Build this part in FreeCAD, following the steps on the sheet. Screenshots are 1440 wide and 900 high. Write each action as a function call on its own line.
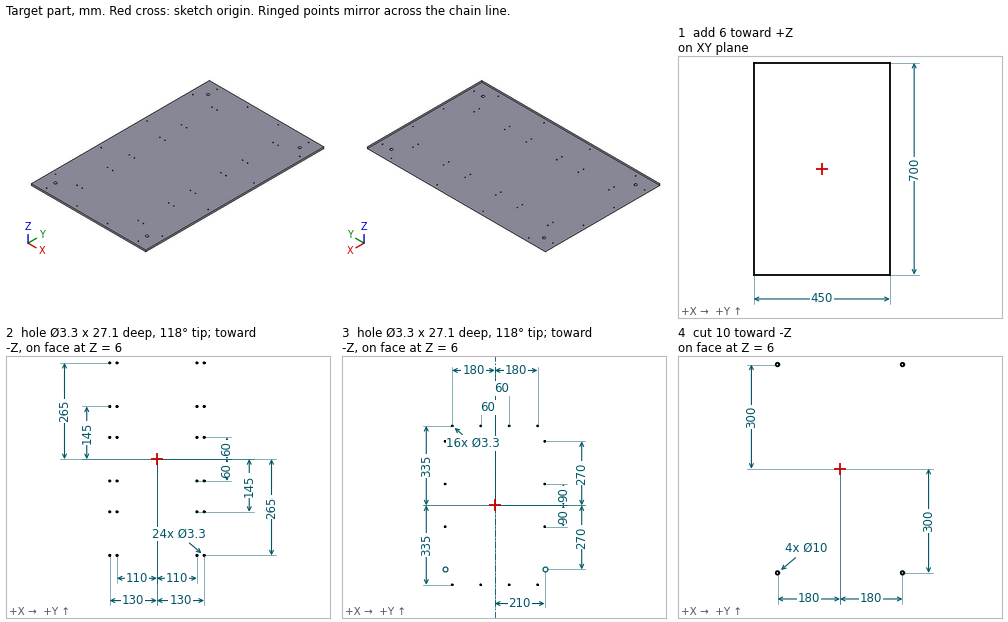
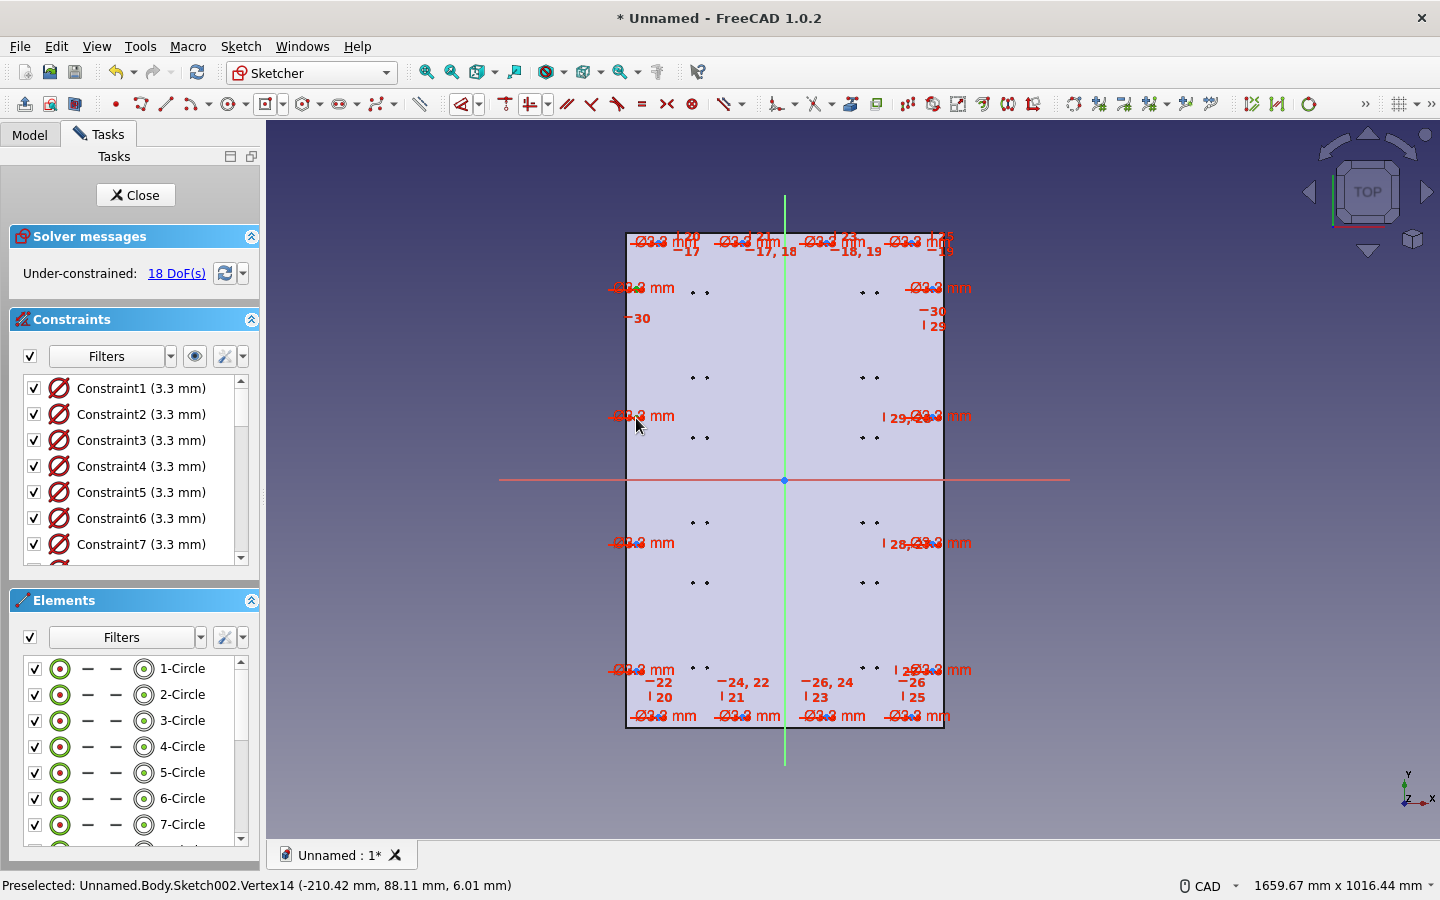
click(548, 104)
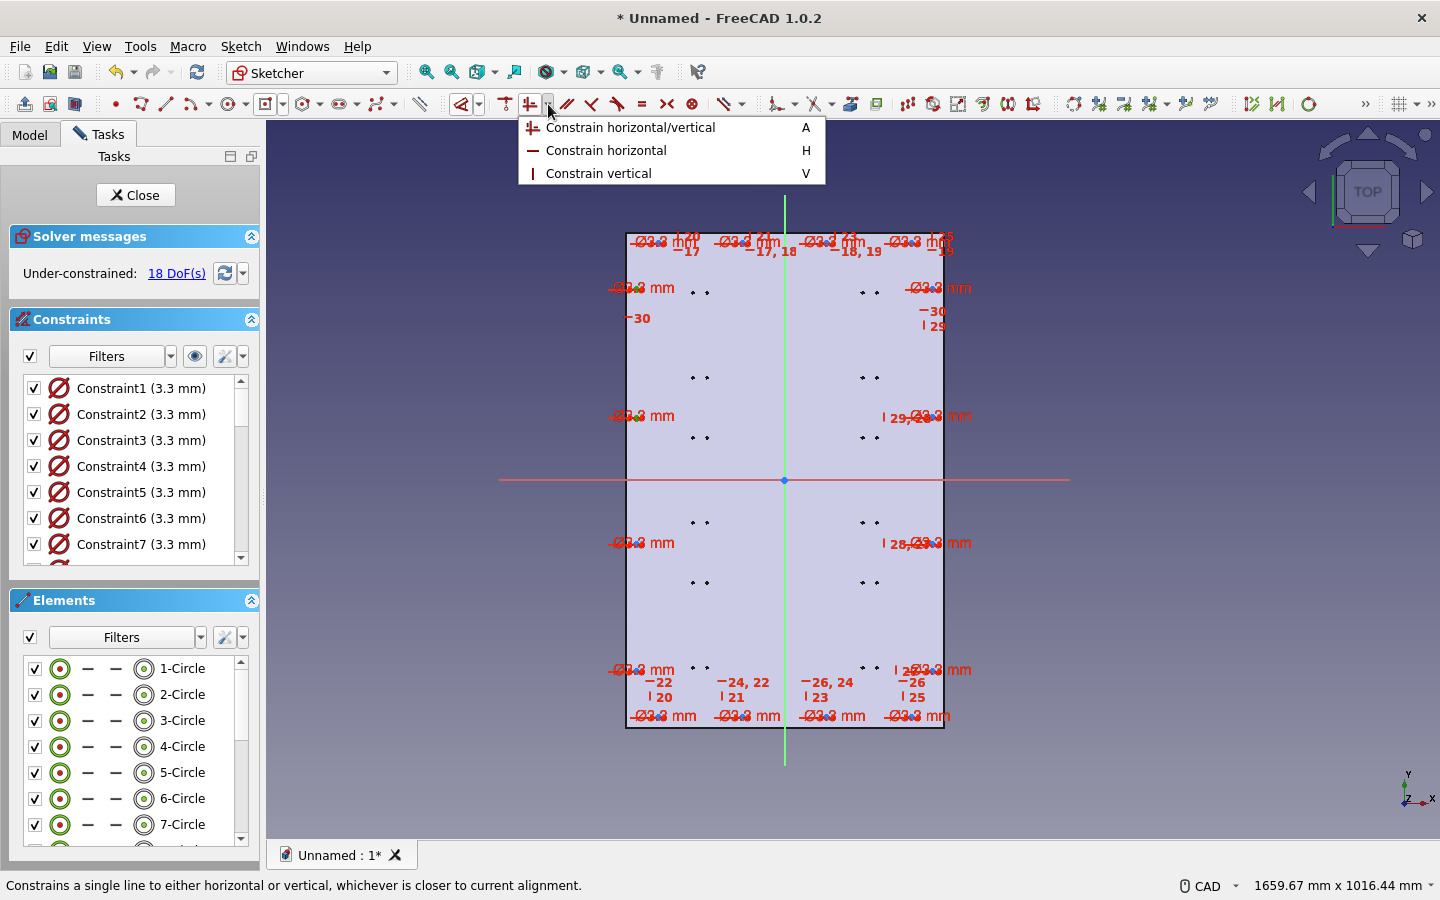
click(672, 174)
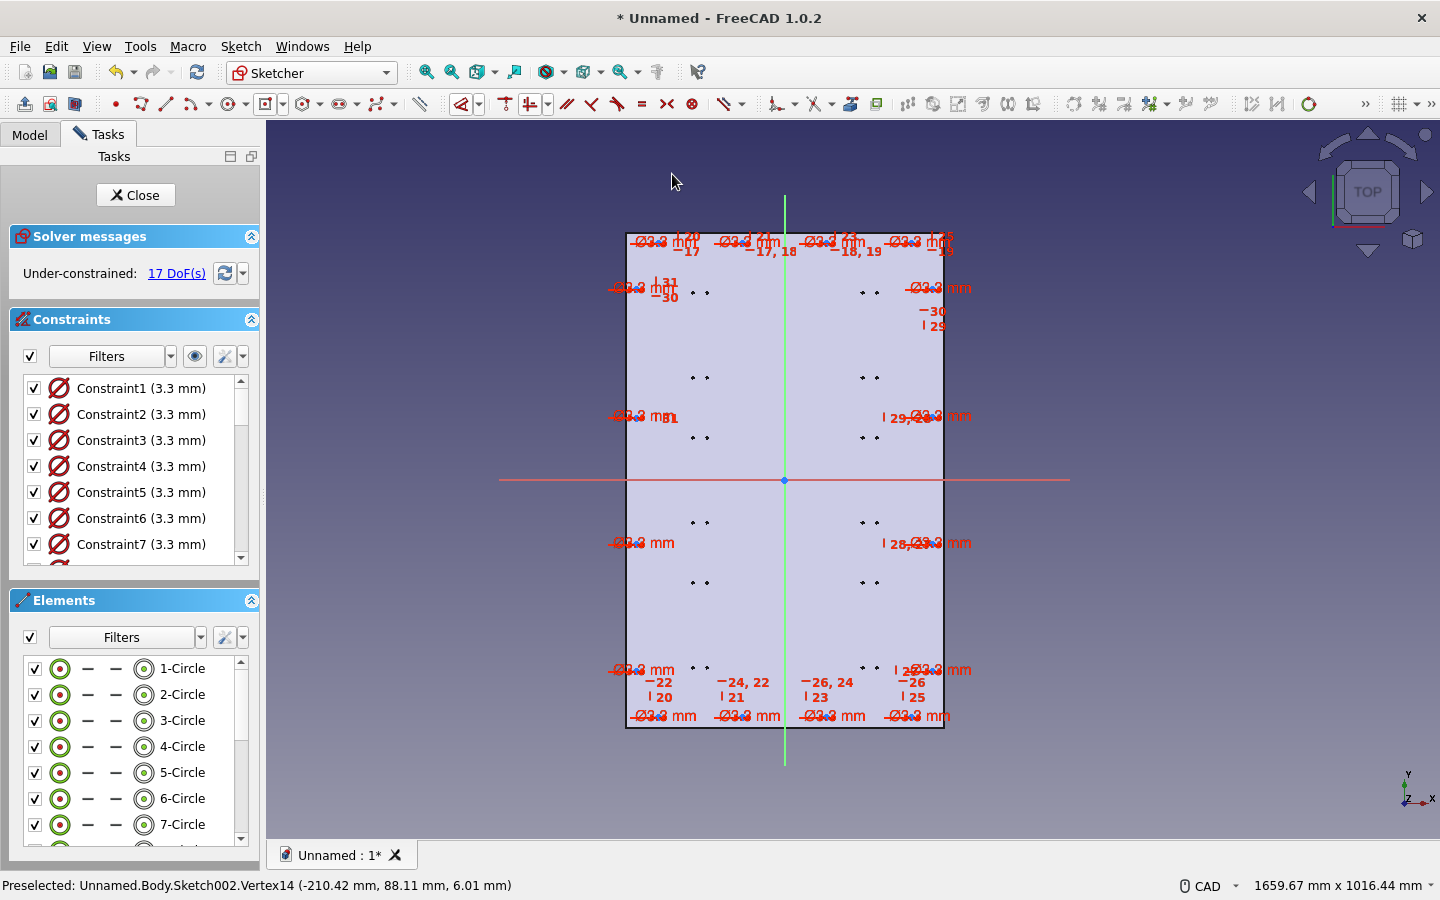
click(933, 418)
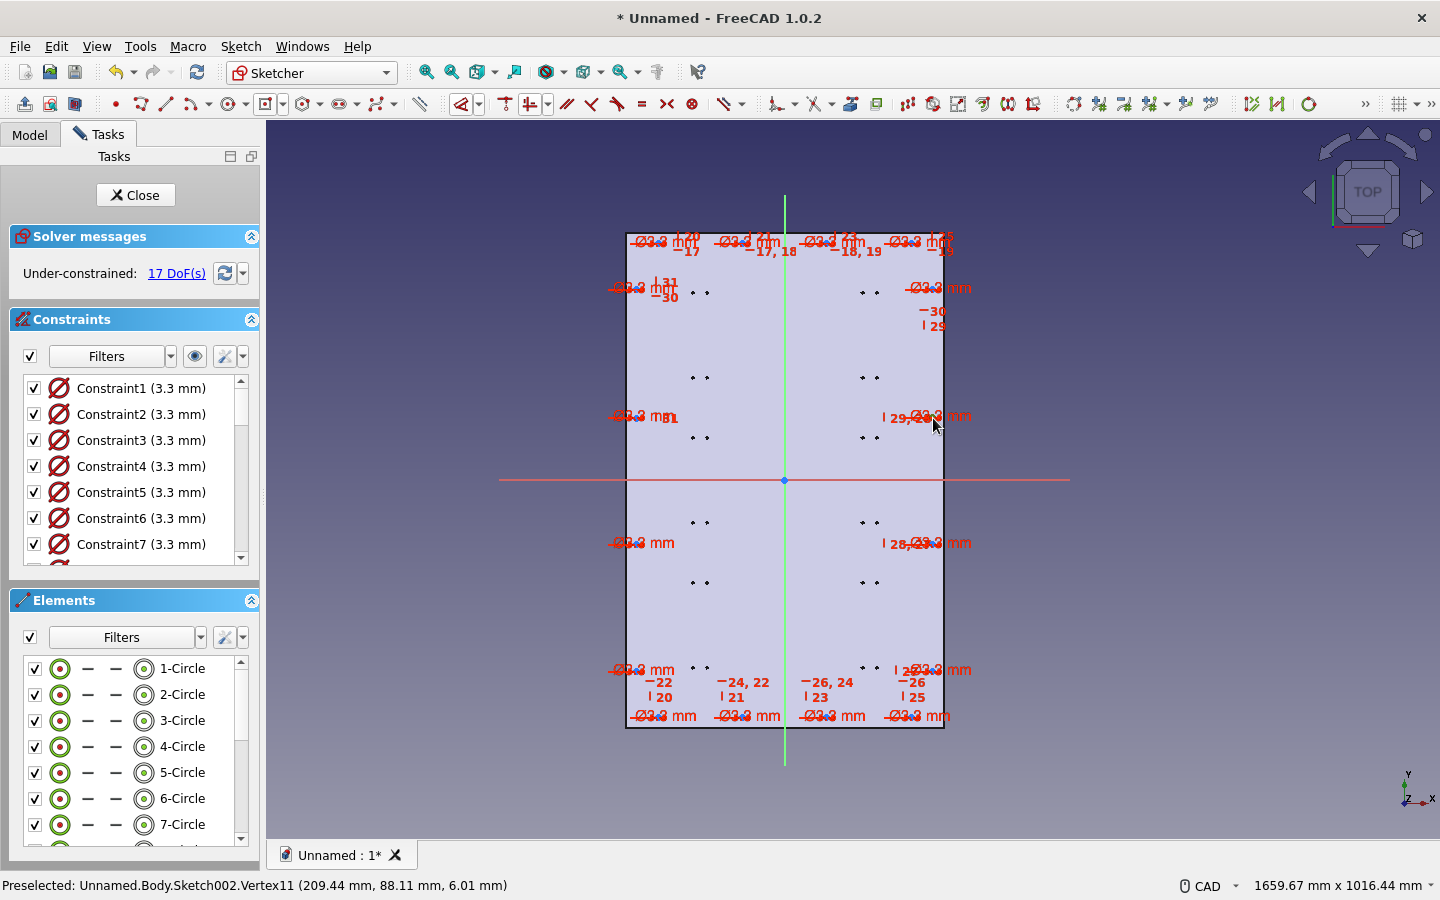
click(636, 418)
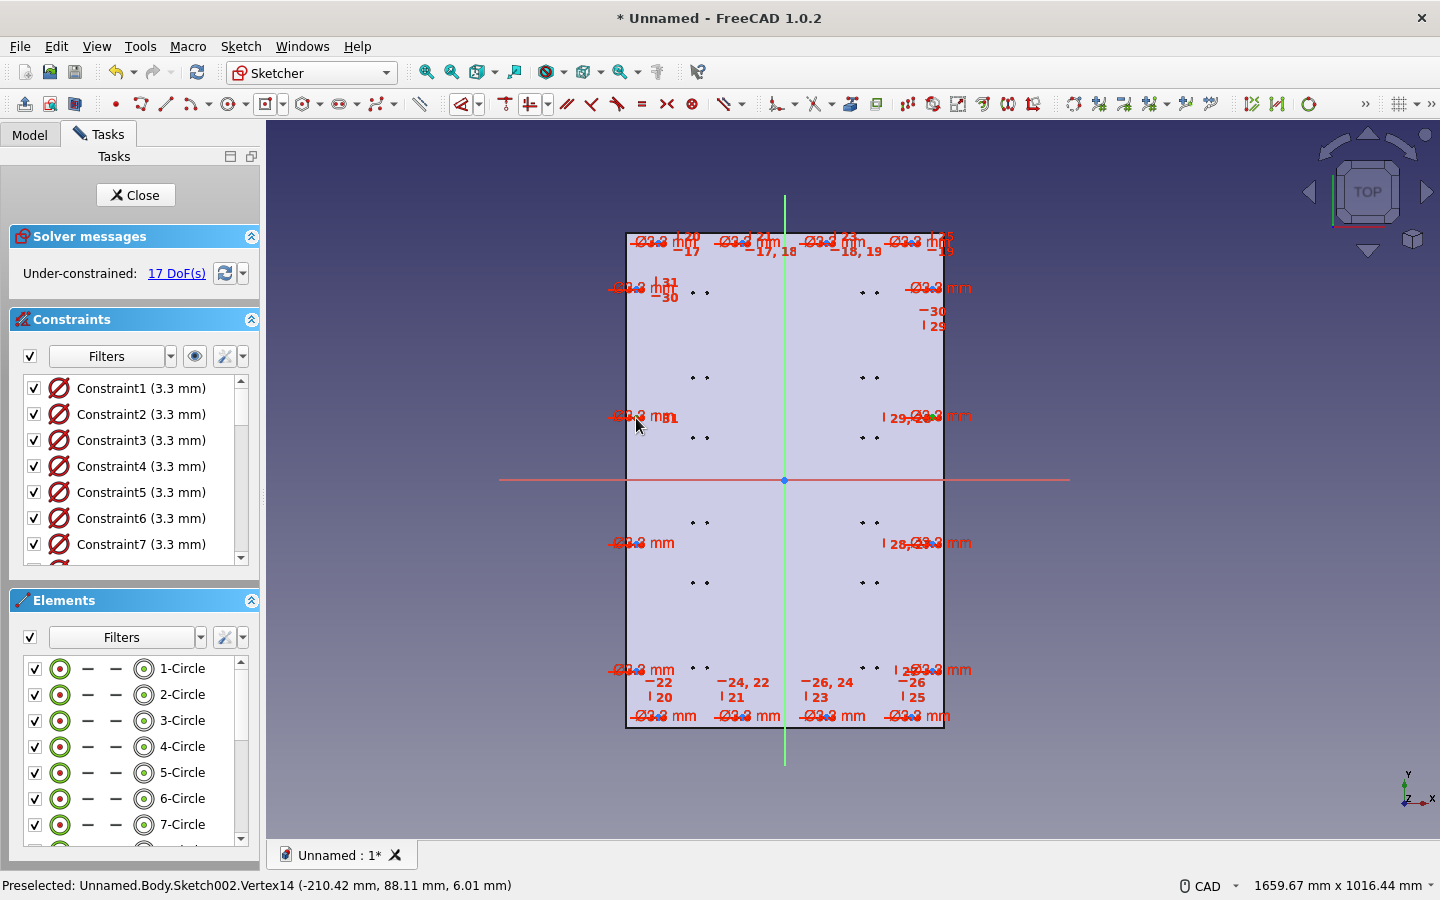
key(h)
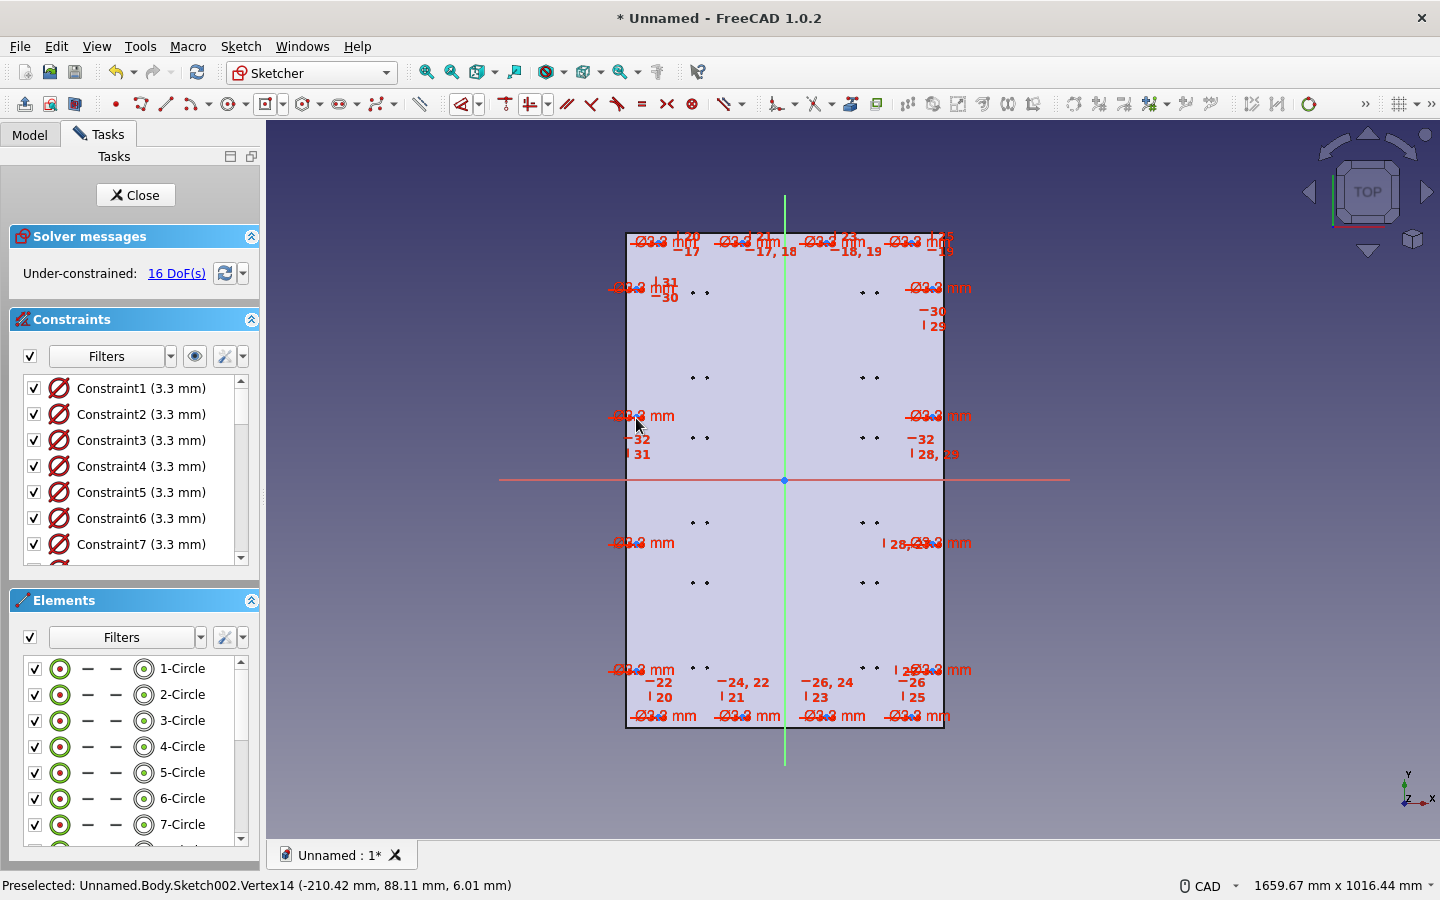
click(636, 418)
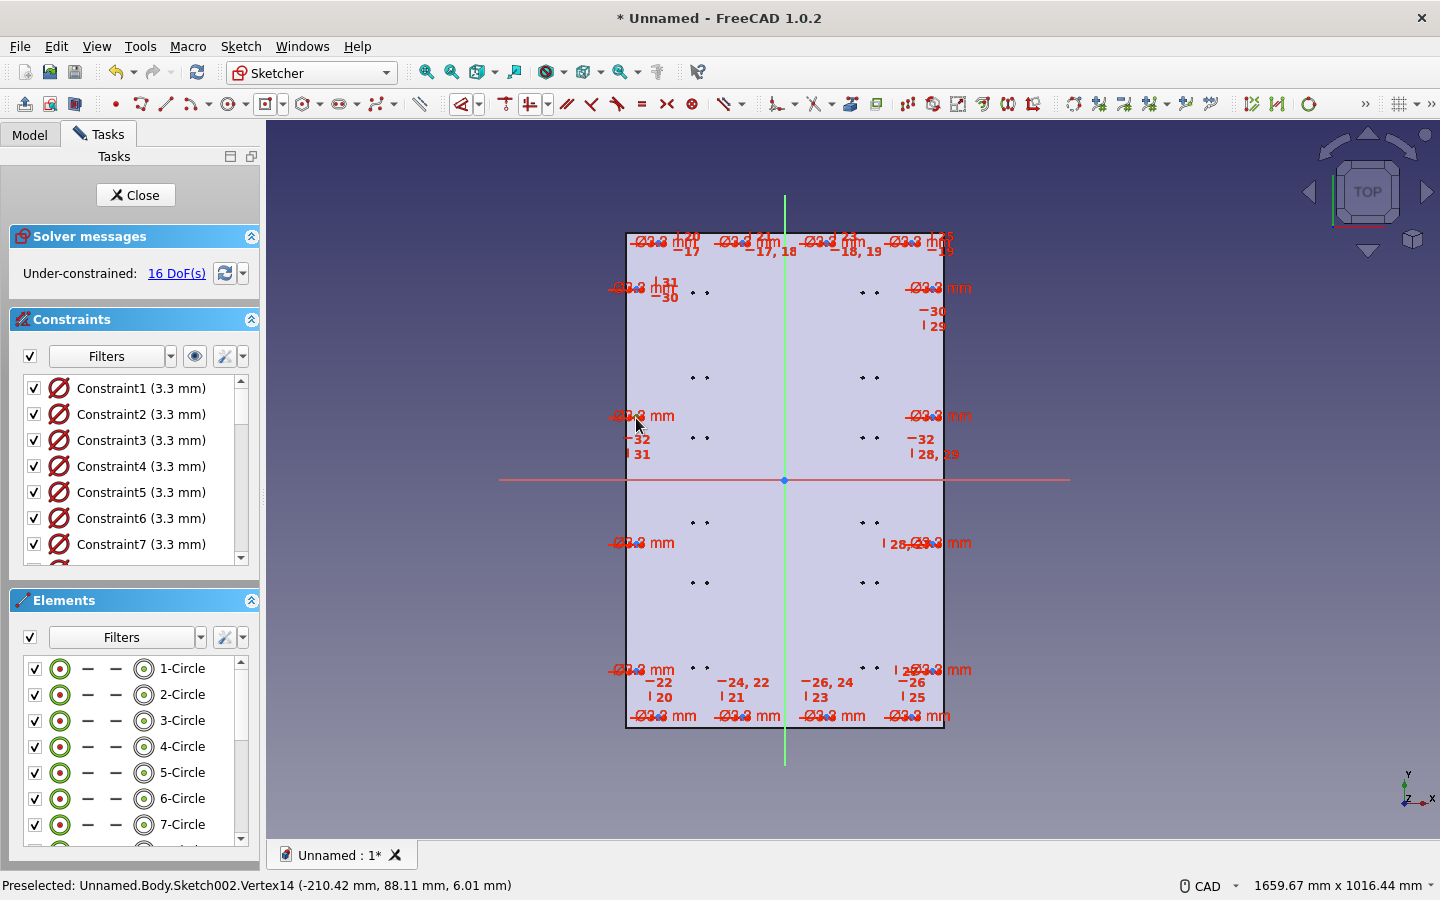
click(636, 545)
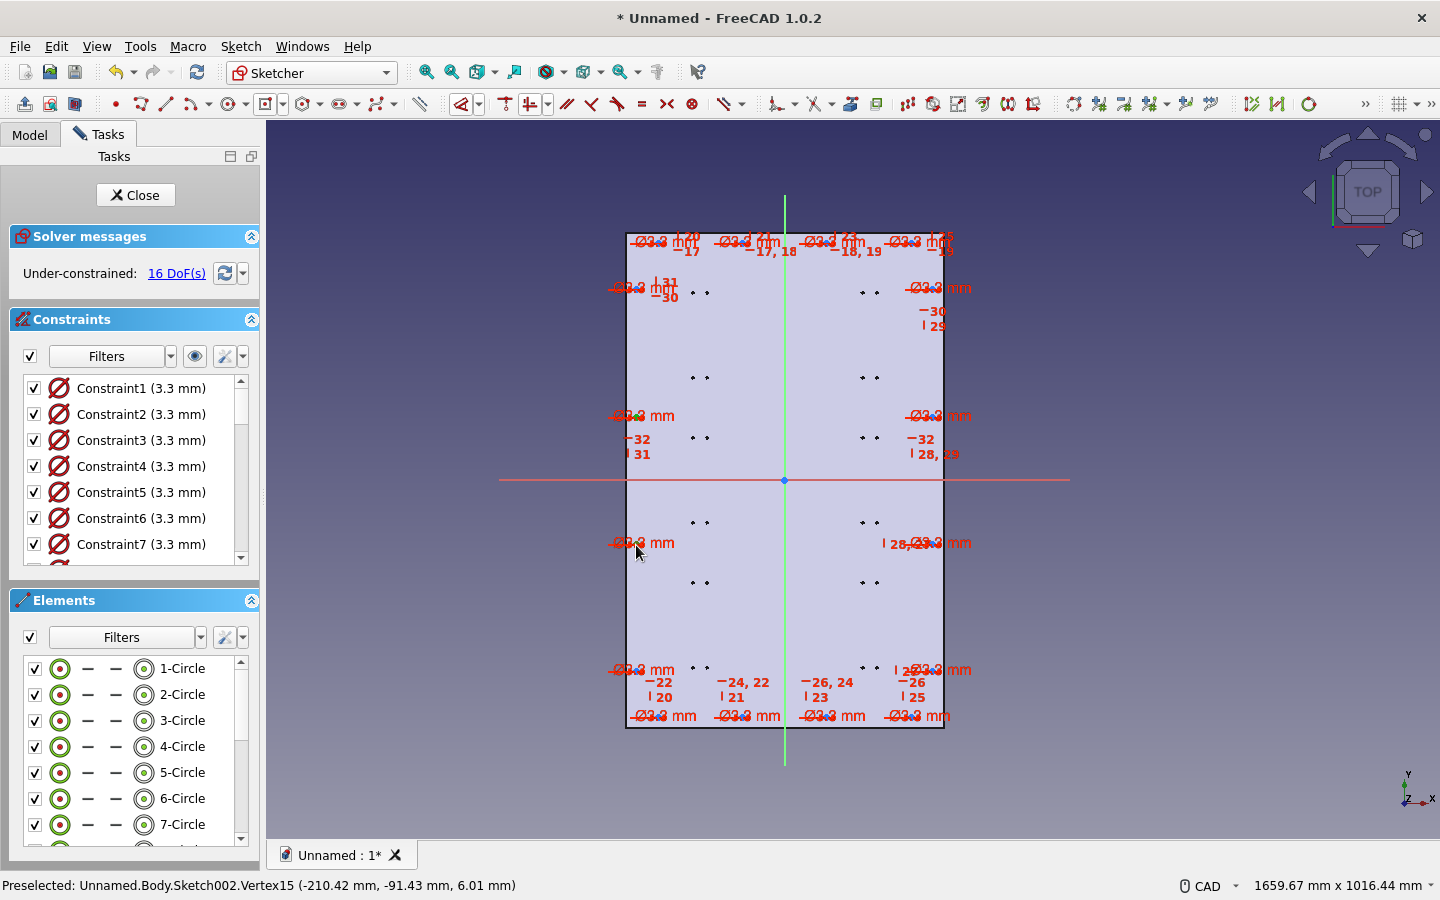
click(548, 104)